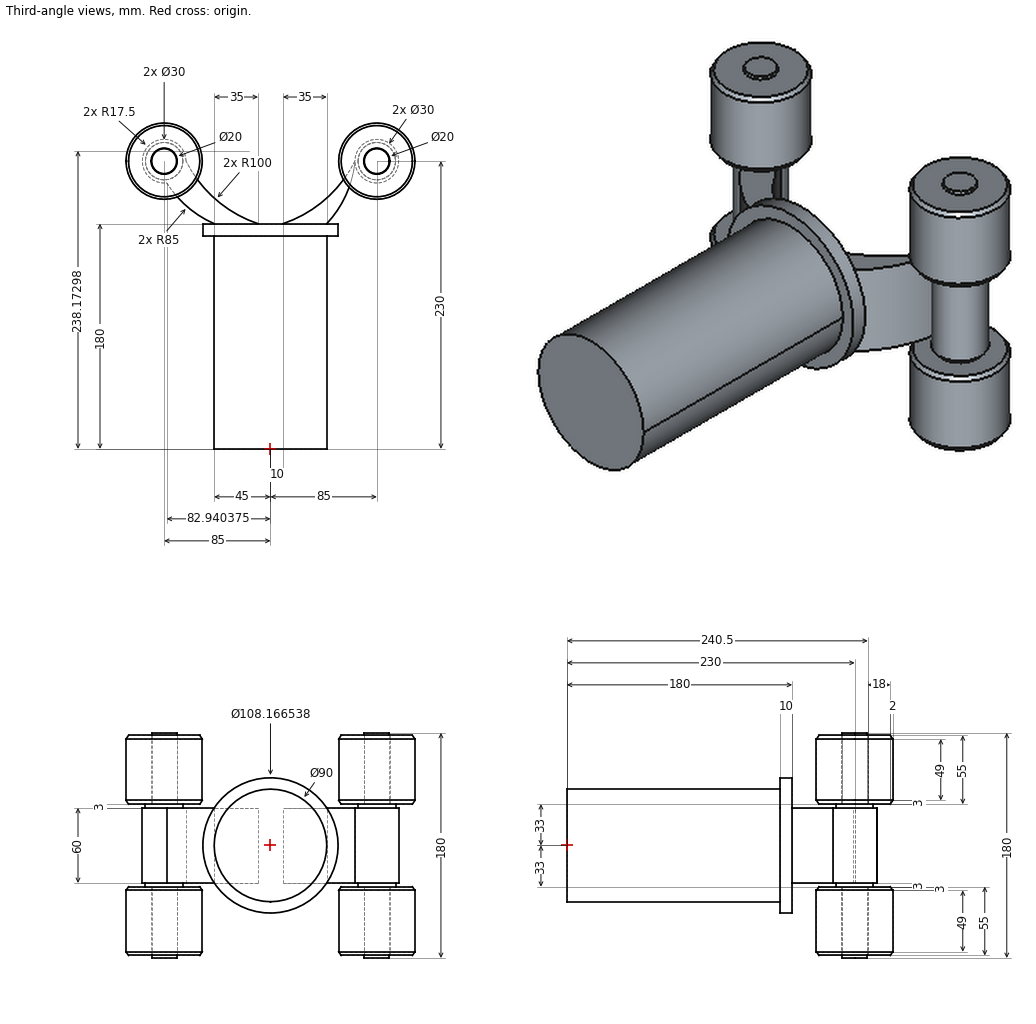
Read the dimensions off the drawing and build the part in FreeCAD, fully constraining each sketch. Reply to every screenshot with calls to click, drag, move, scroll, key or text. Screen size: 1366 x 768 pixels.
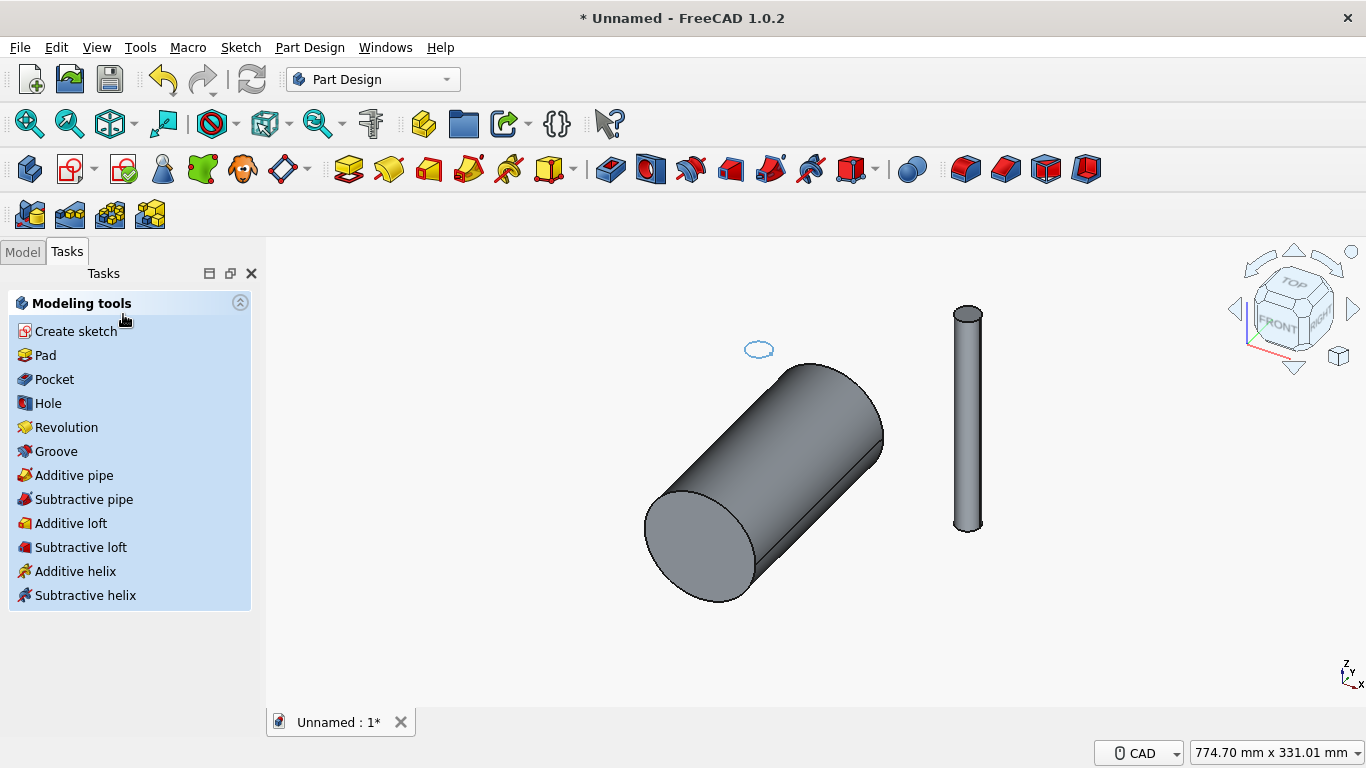
click(350, 170)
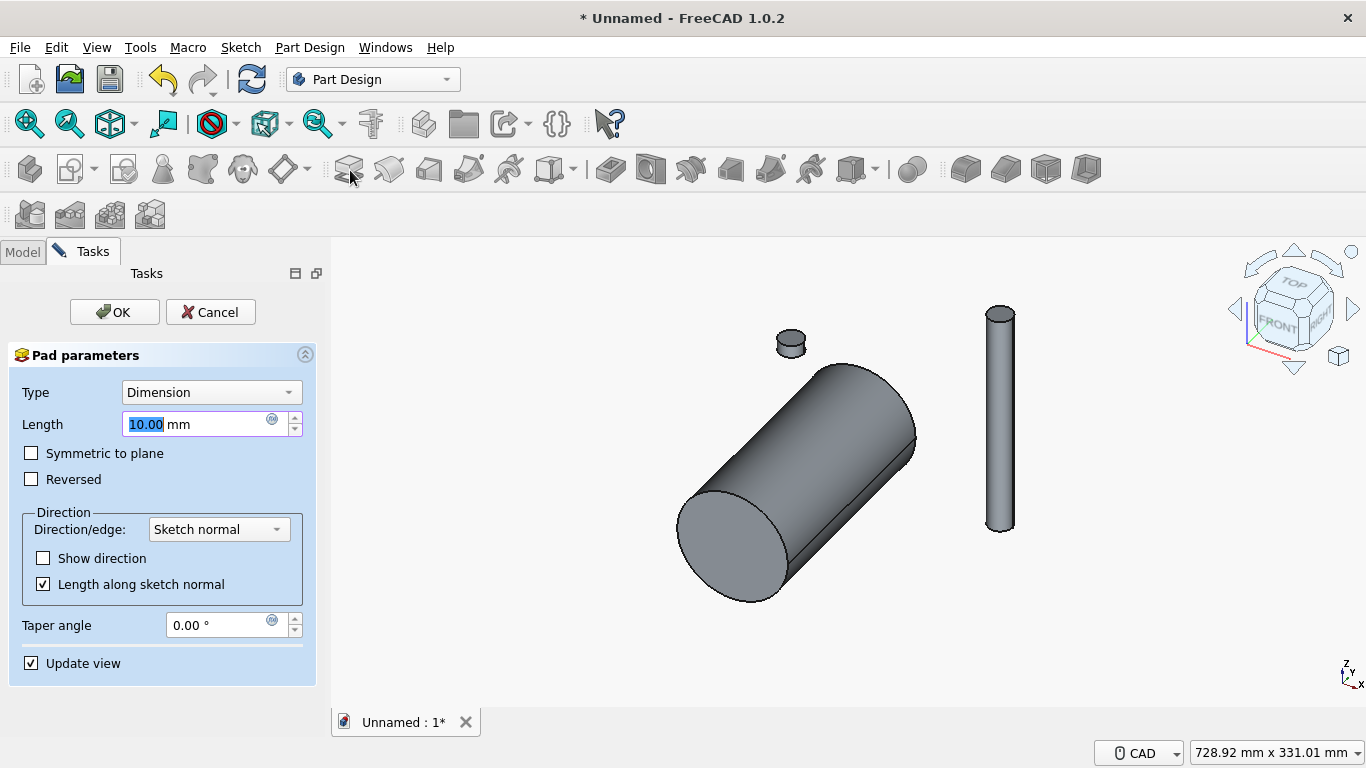
text(180)
key(Tab)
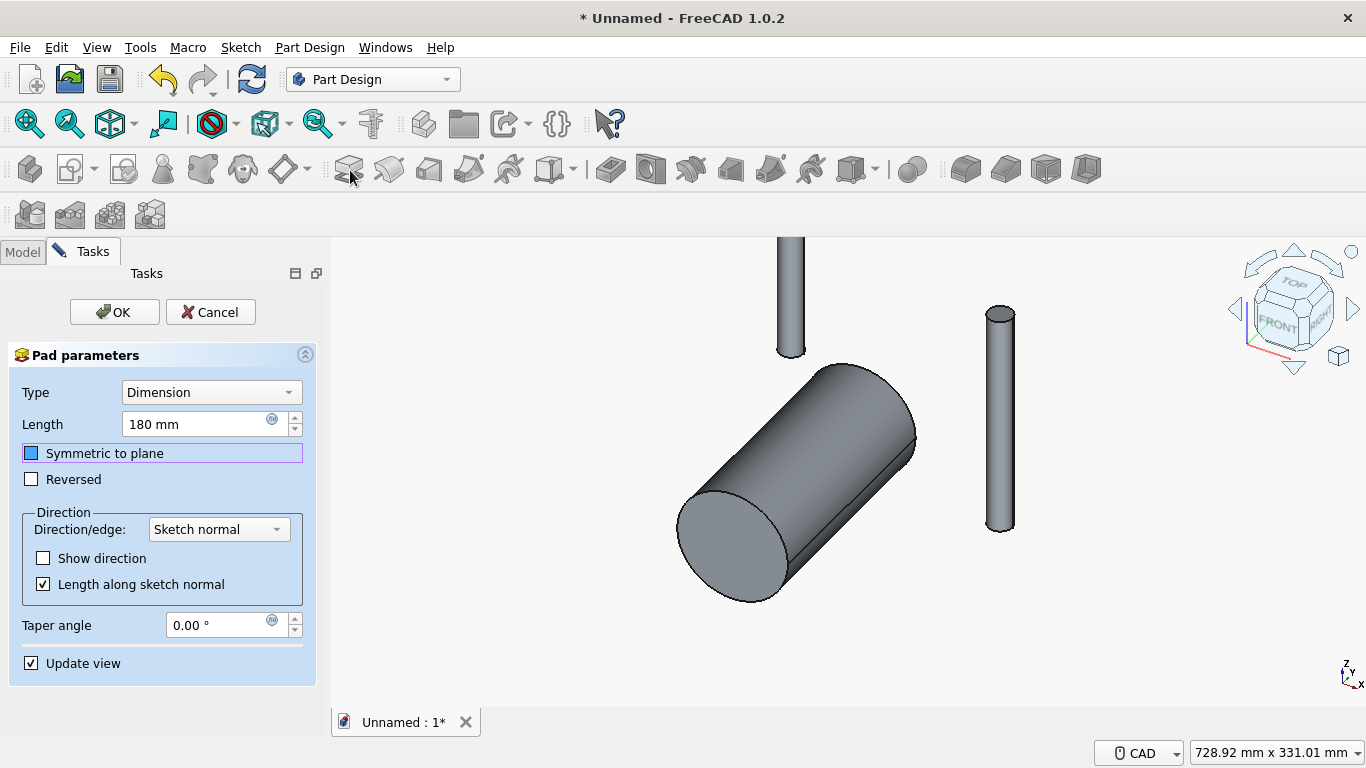
click(30, 453)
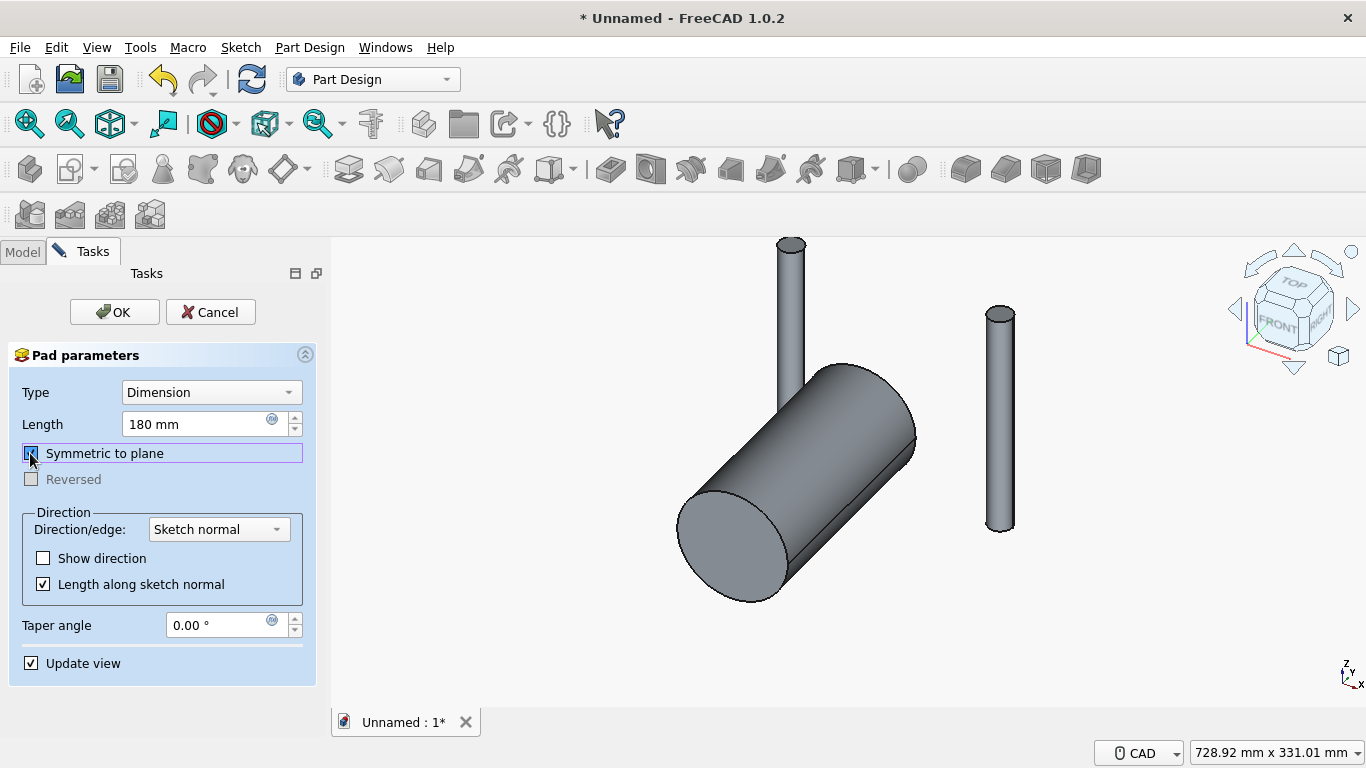
click(115, 312)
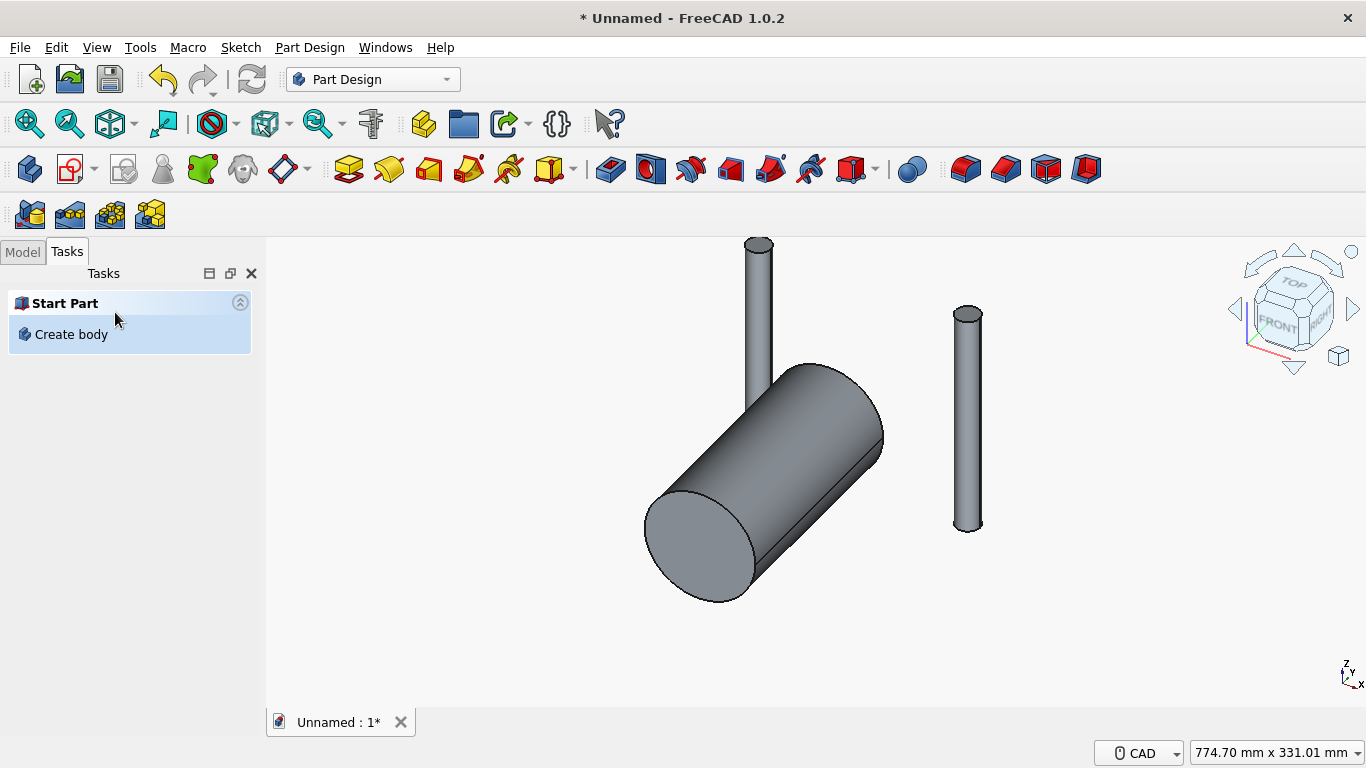
click(30, 124)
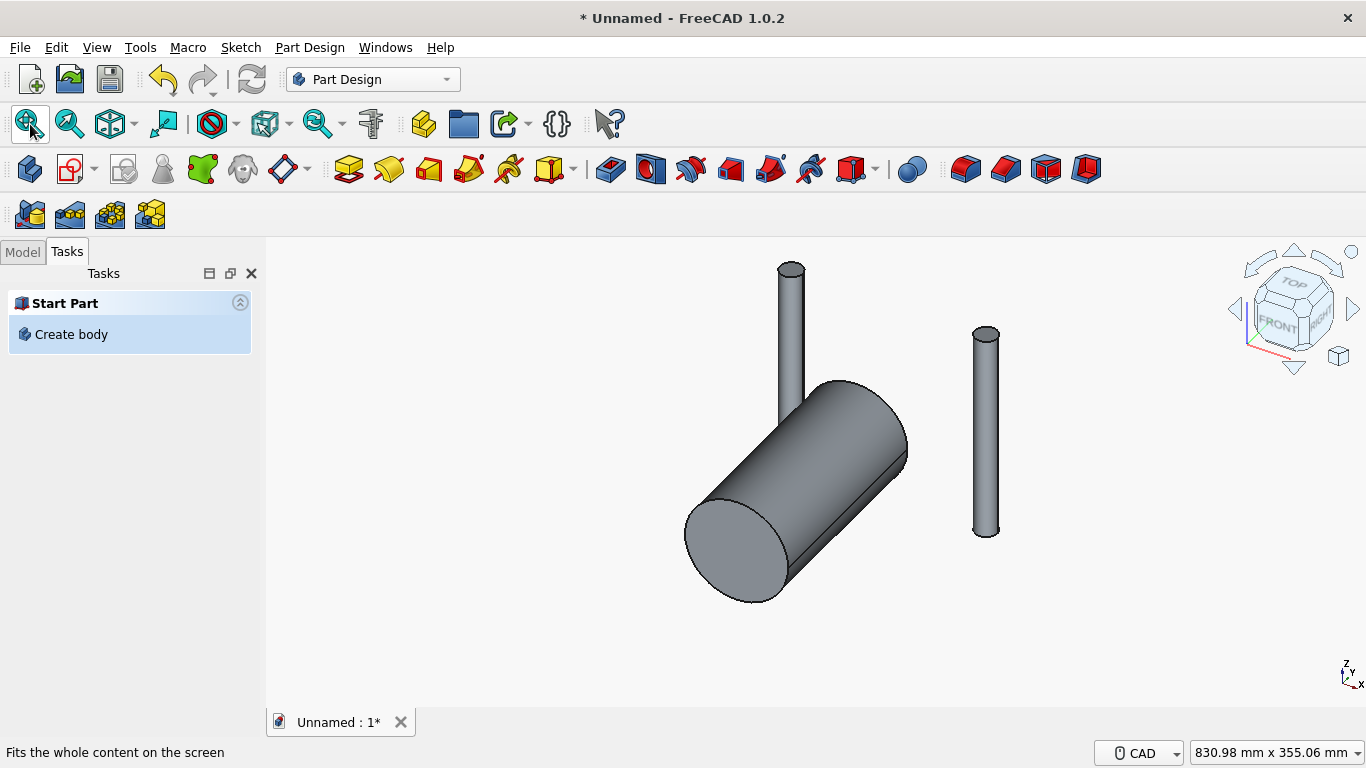
click(23, 251)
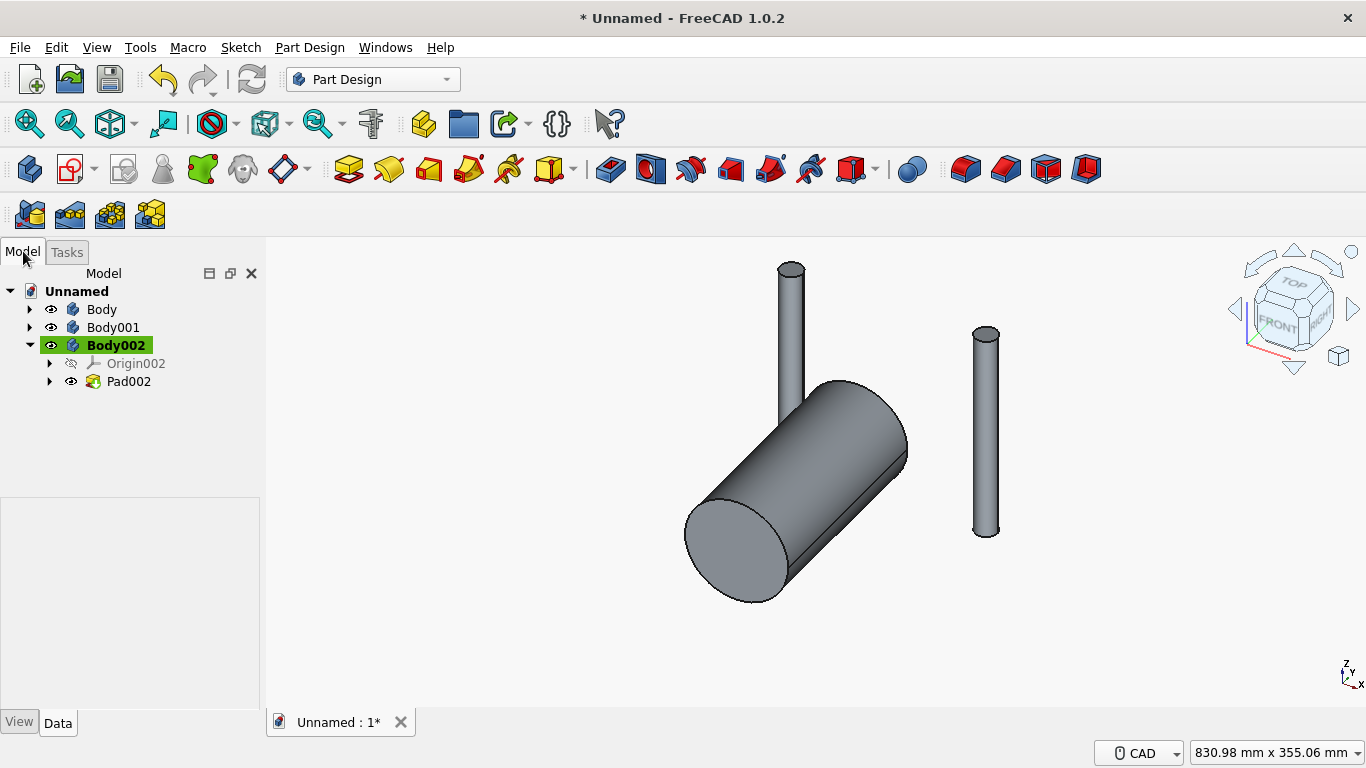
double_click(96, 309)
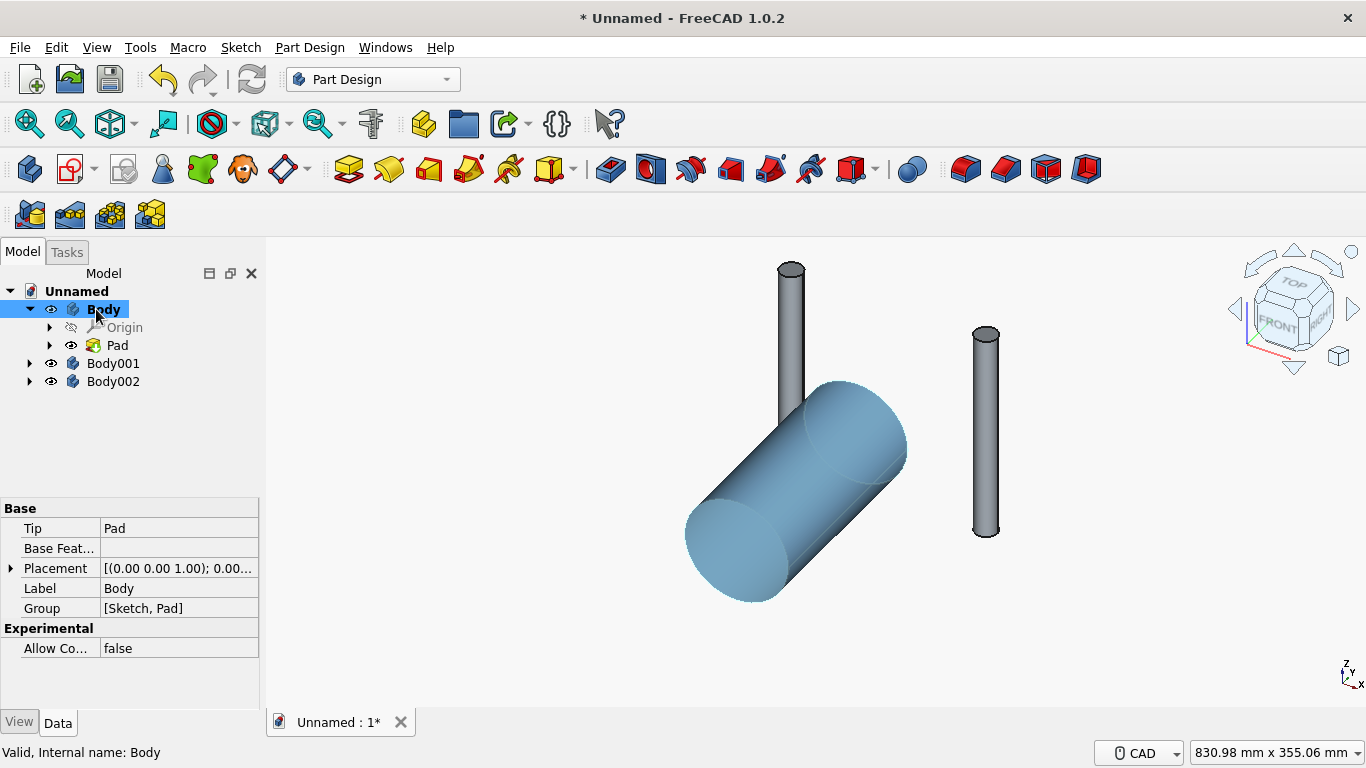
click(96, 309)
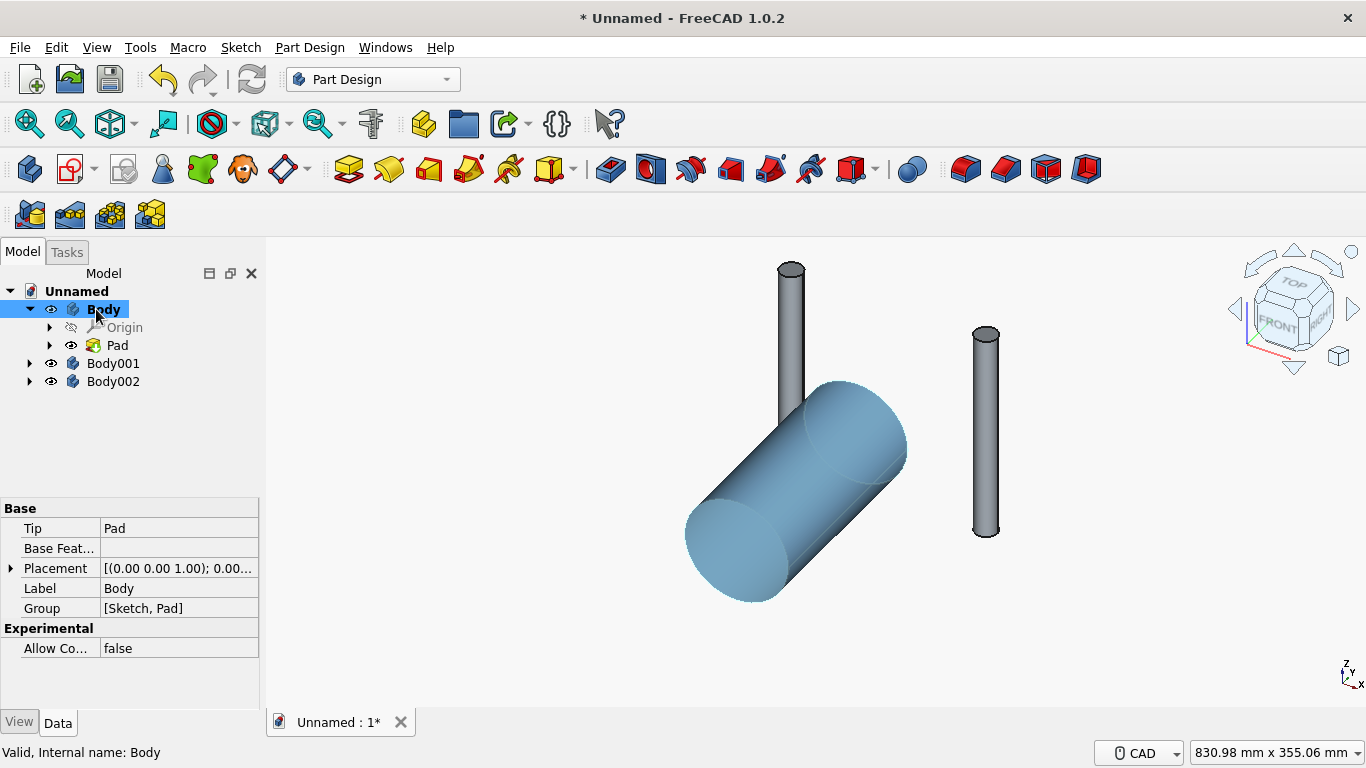
click(146, 648)